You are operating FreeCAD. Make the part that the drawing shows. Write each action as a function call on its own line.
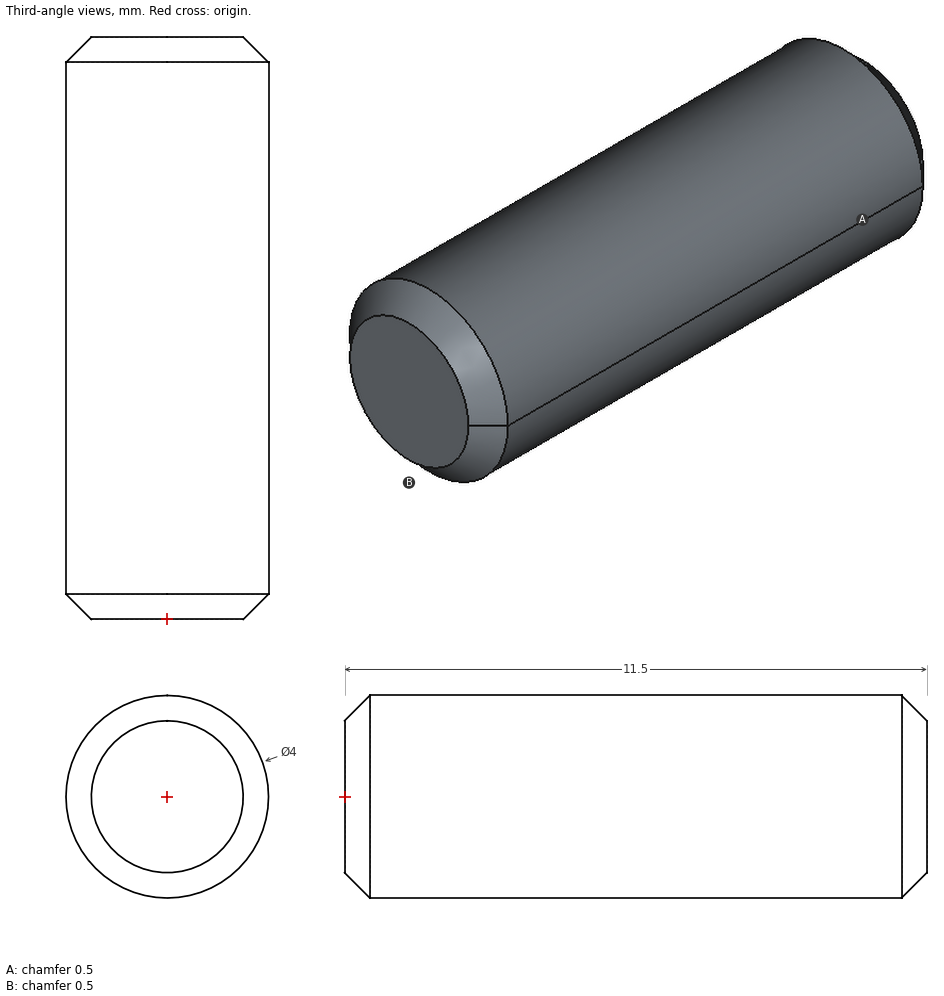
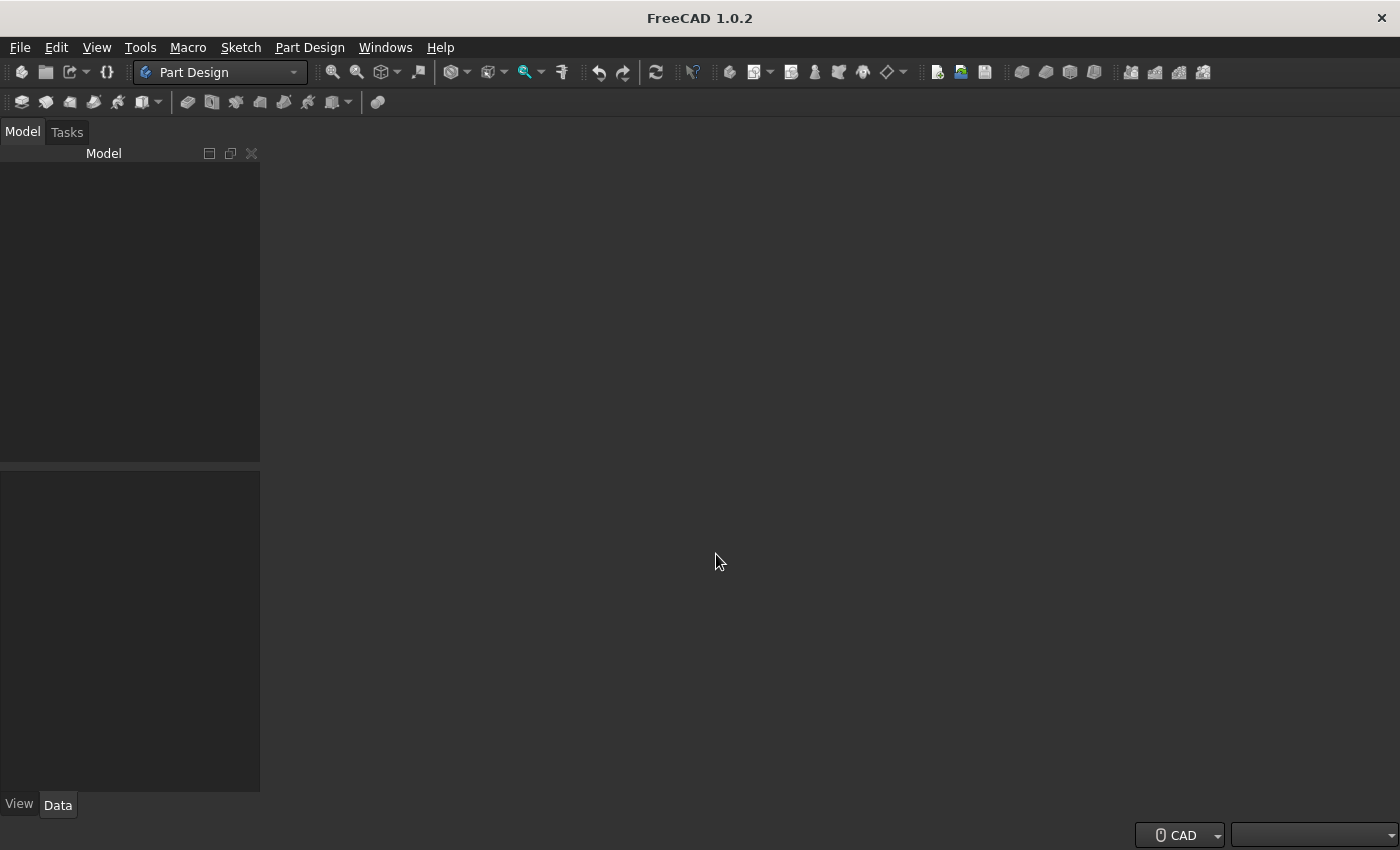
click(938, 72)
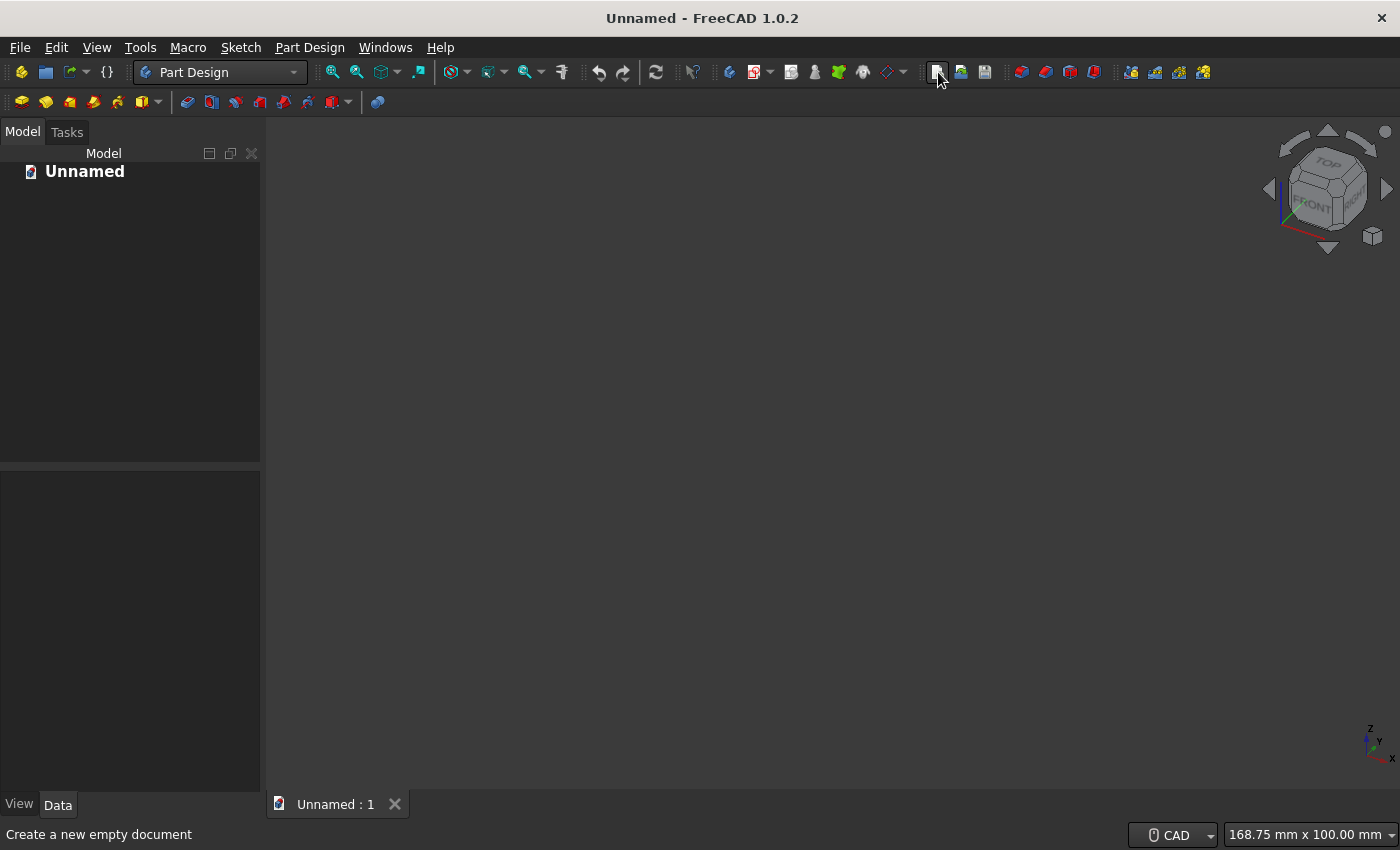
click(754, 72)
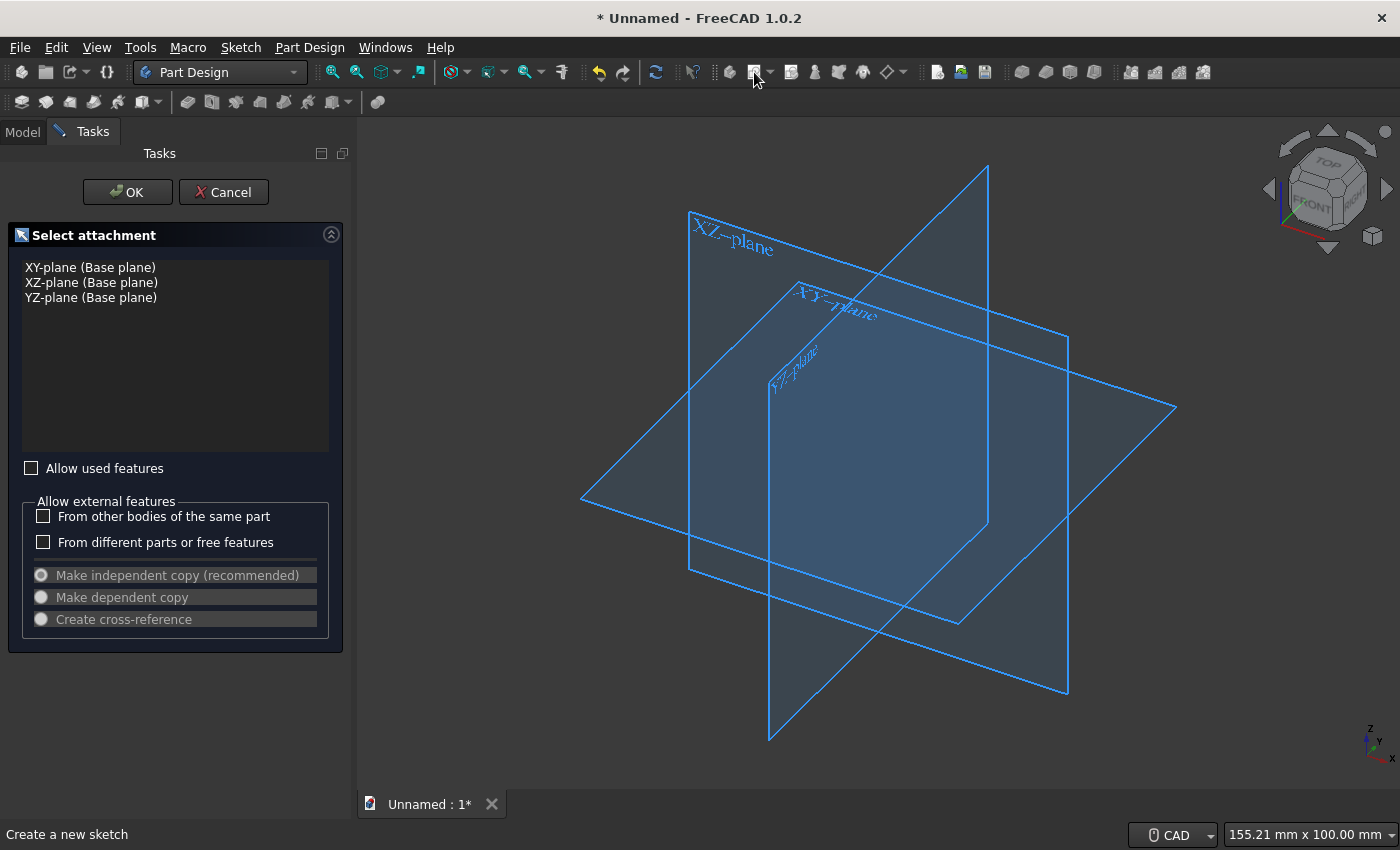
click(82, 282)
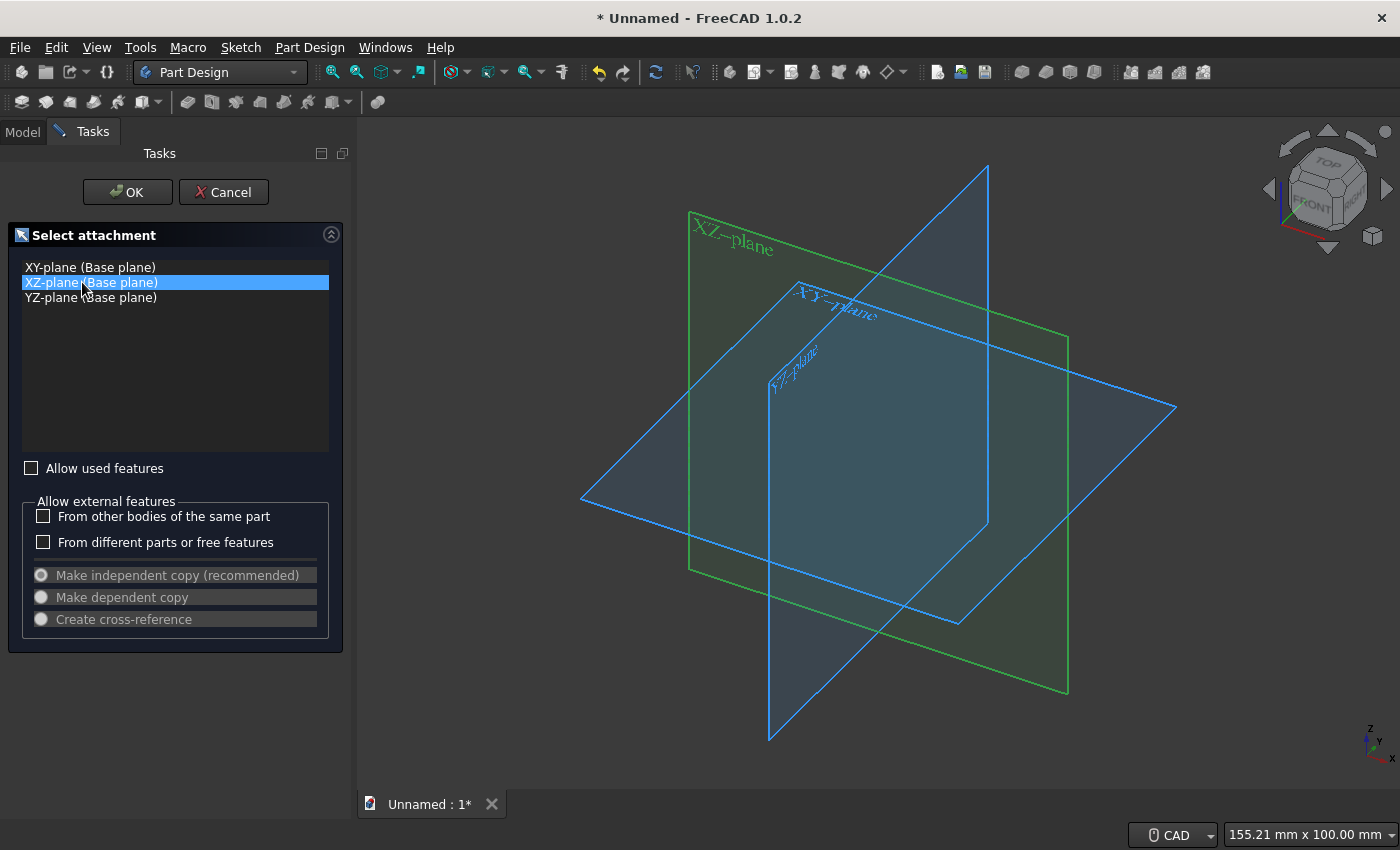
click(128, 192)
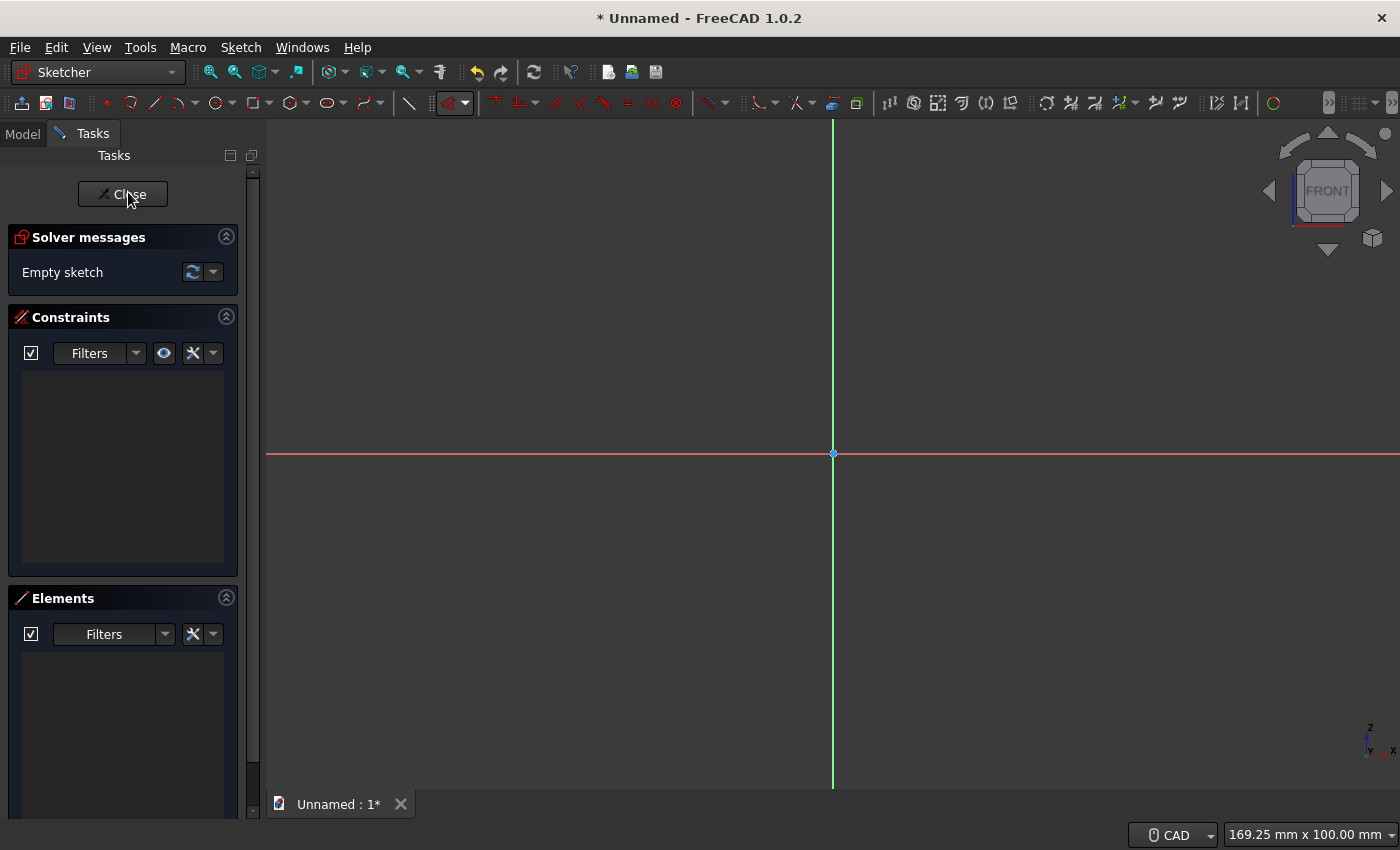
scroll(837, 454, up, 14)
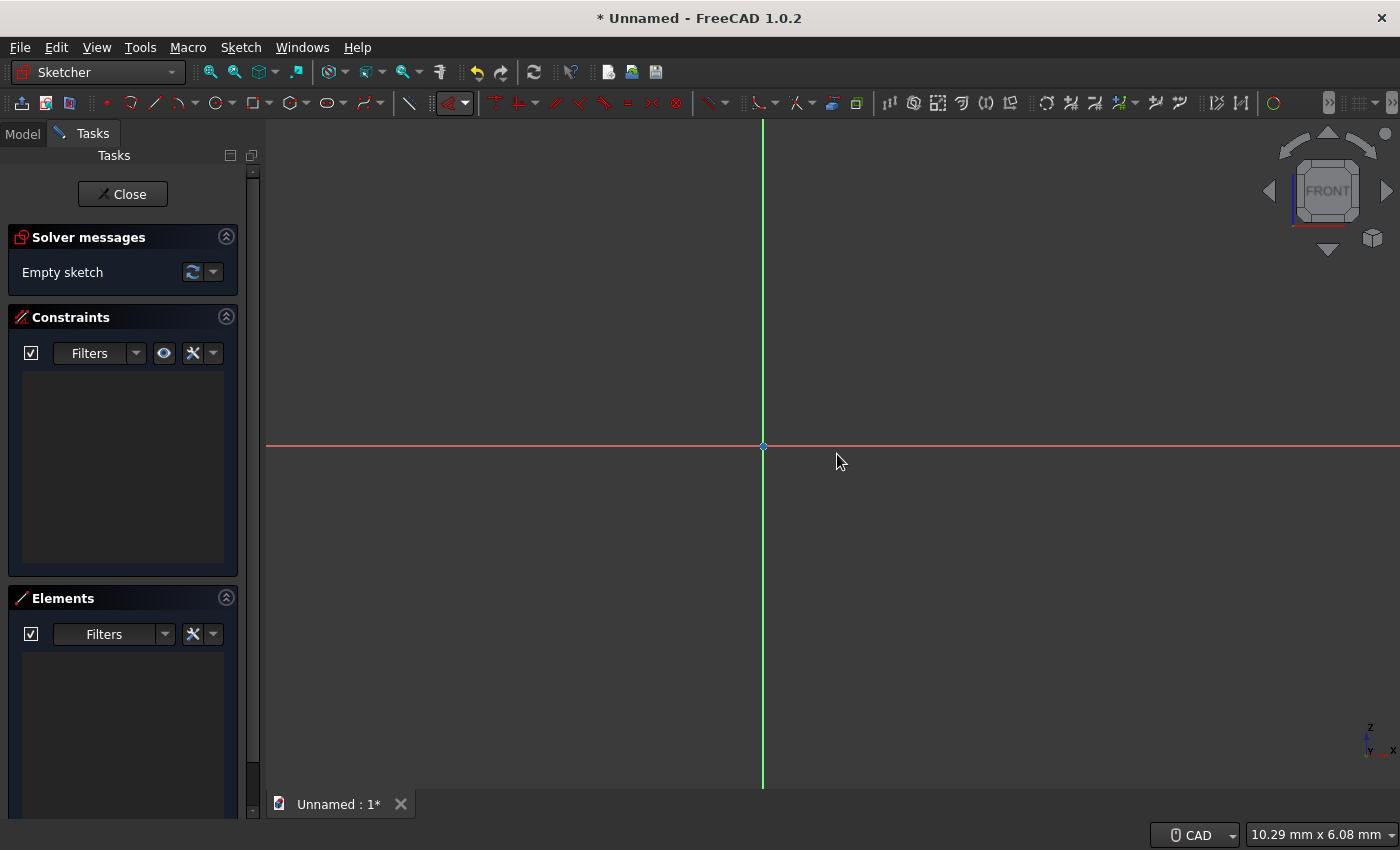
click(216, 104)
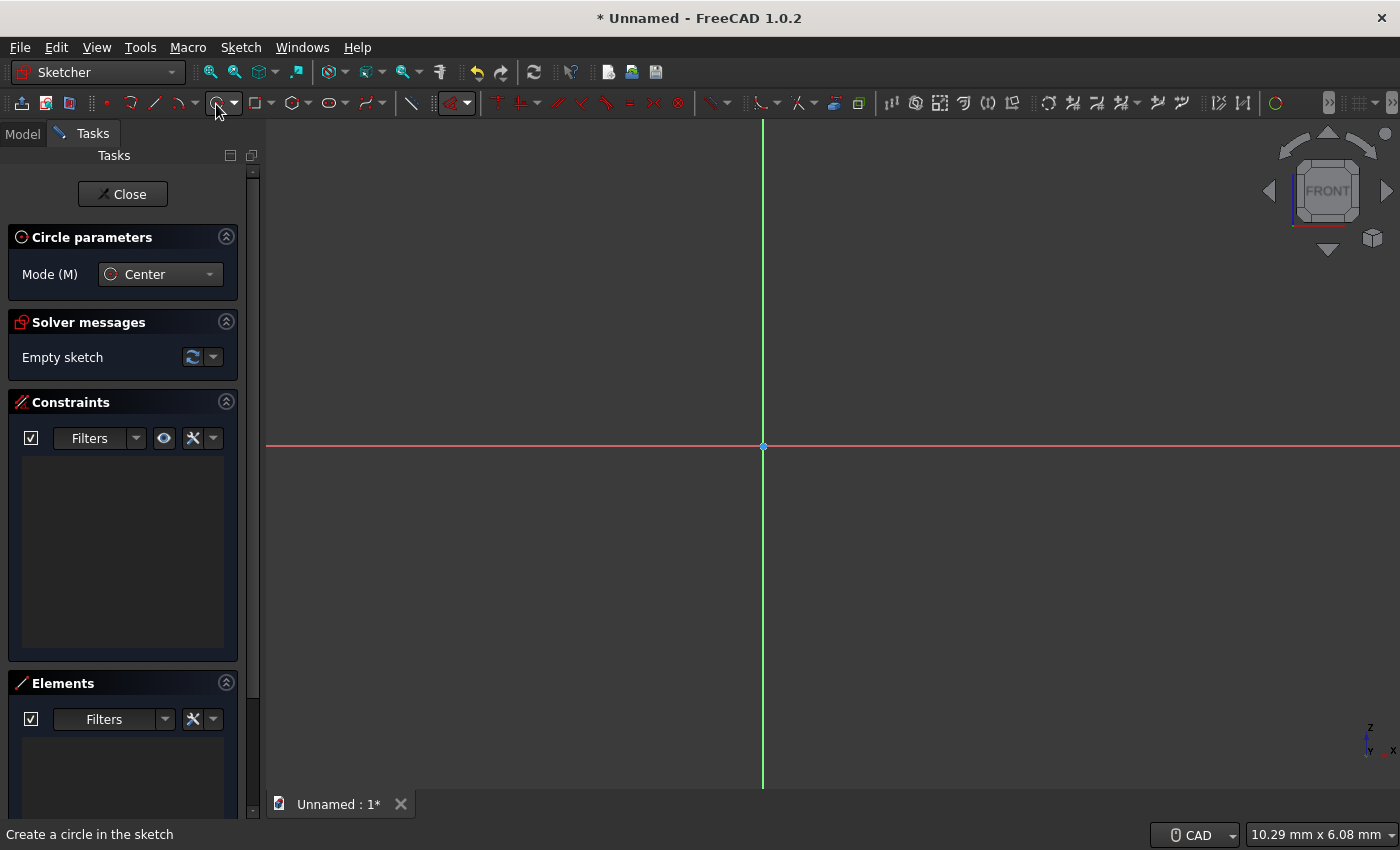
click(763, 446)
move(919, 290)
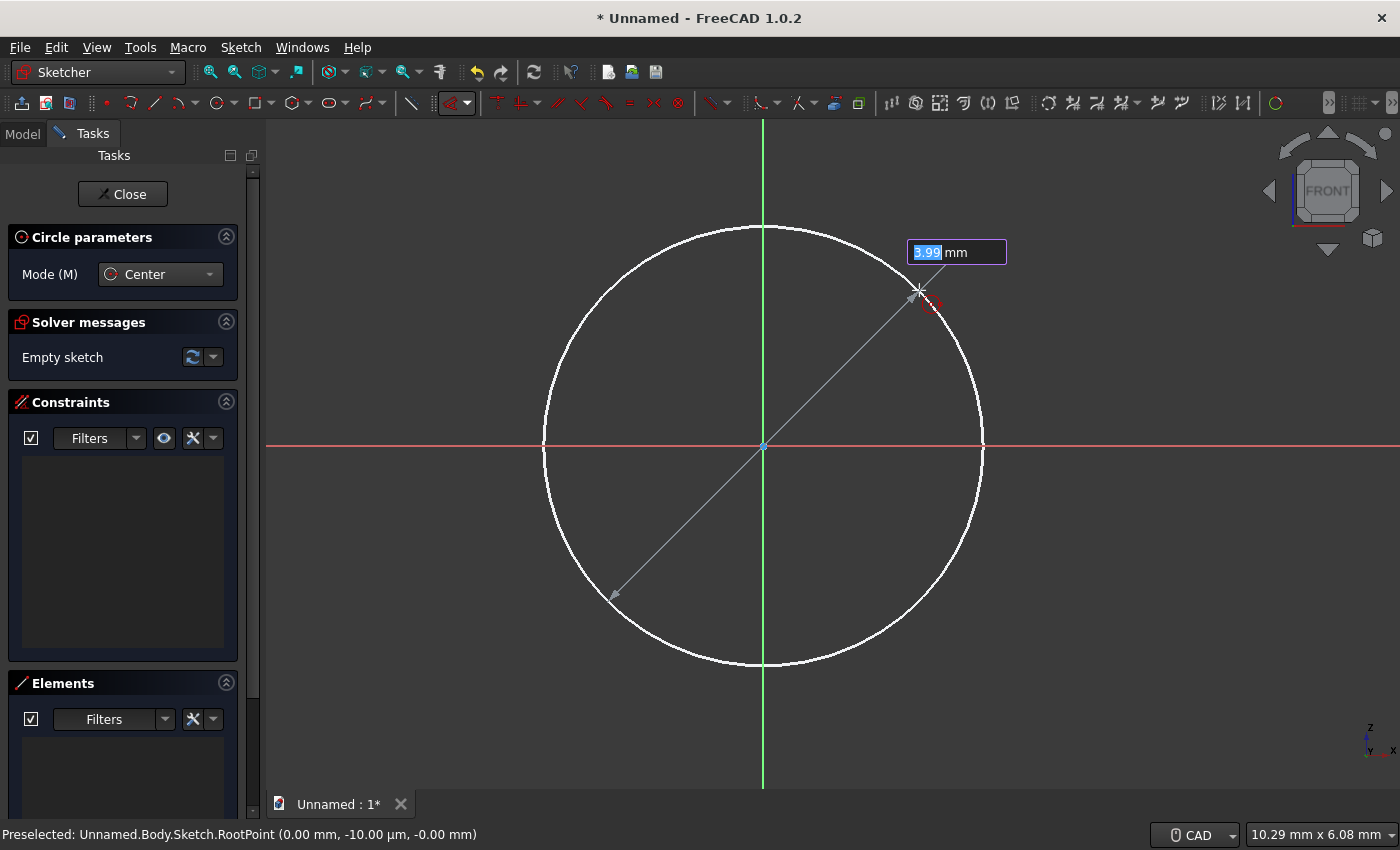
text(4)
key(Return)
key(Escape)